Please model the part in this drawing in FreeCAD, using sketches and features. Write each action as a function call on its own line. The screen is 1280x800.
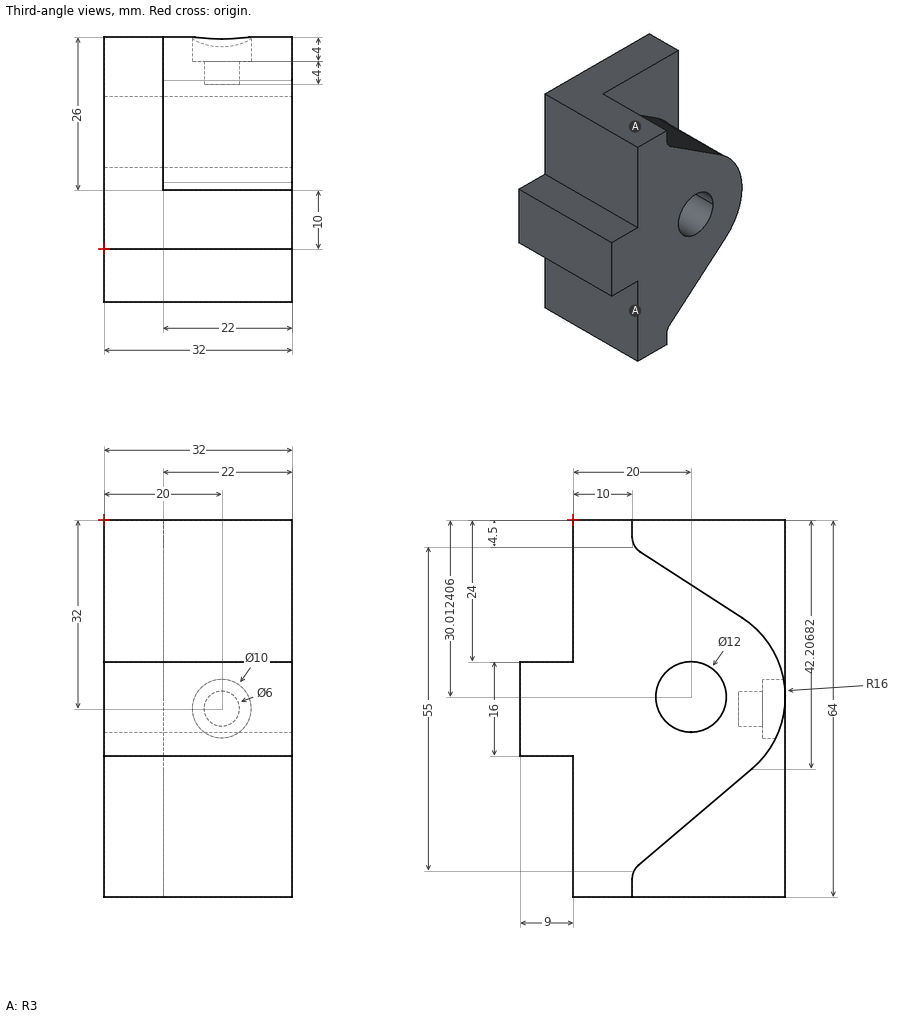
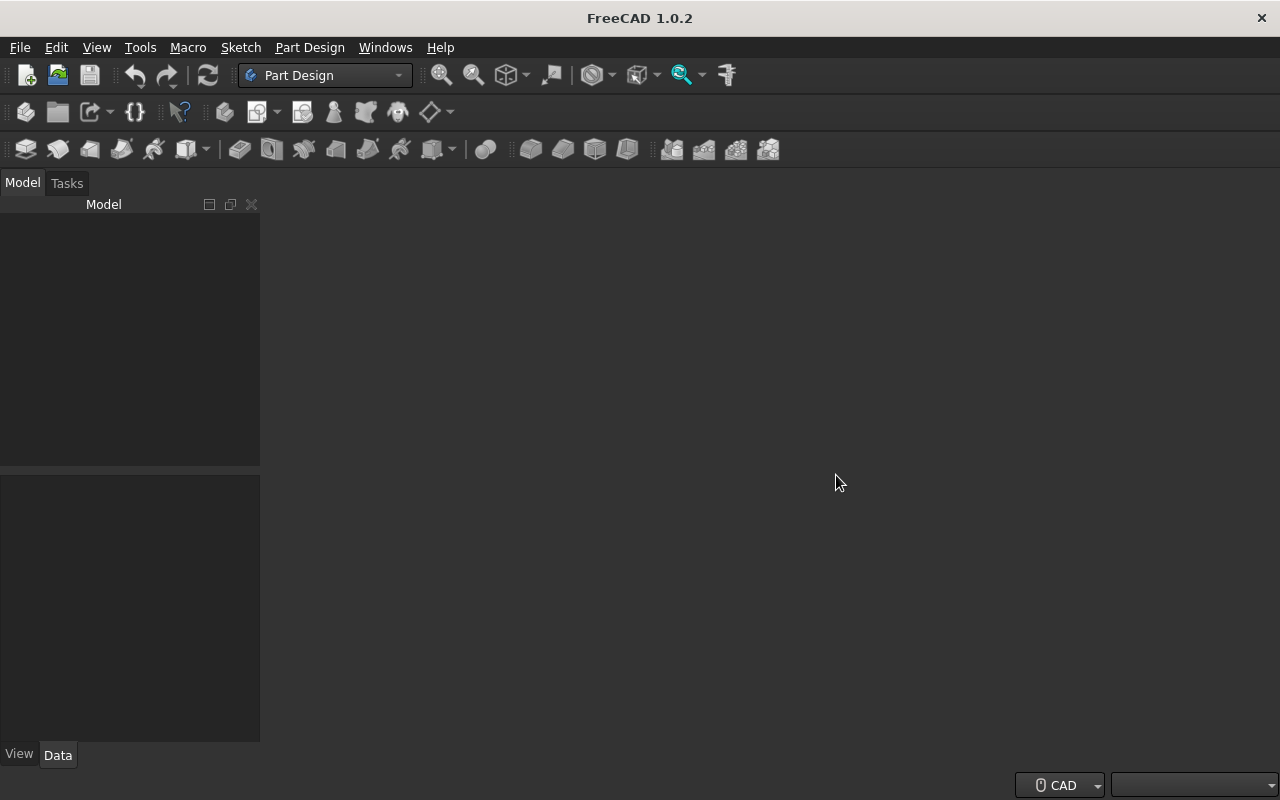
key(ctrl+n)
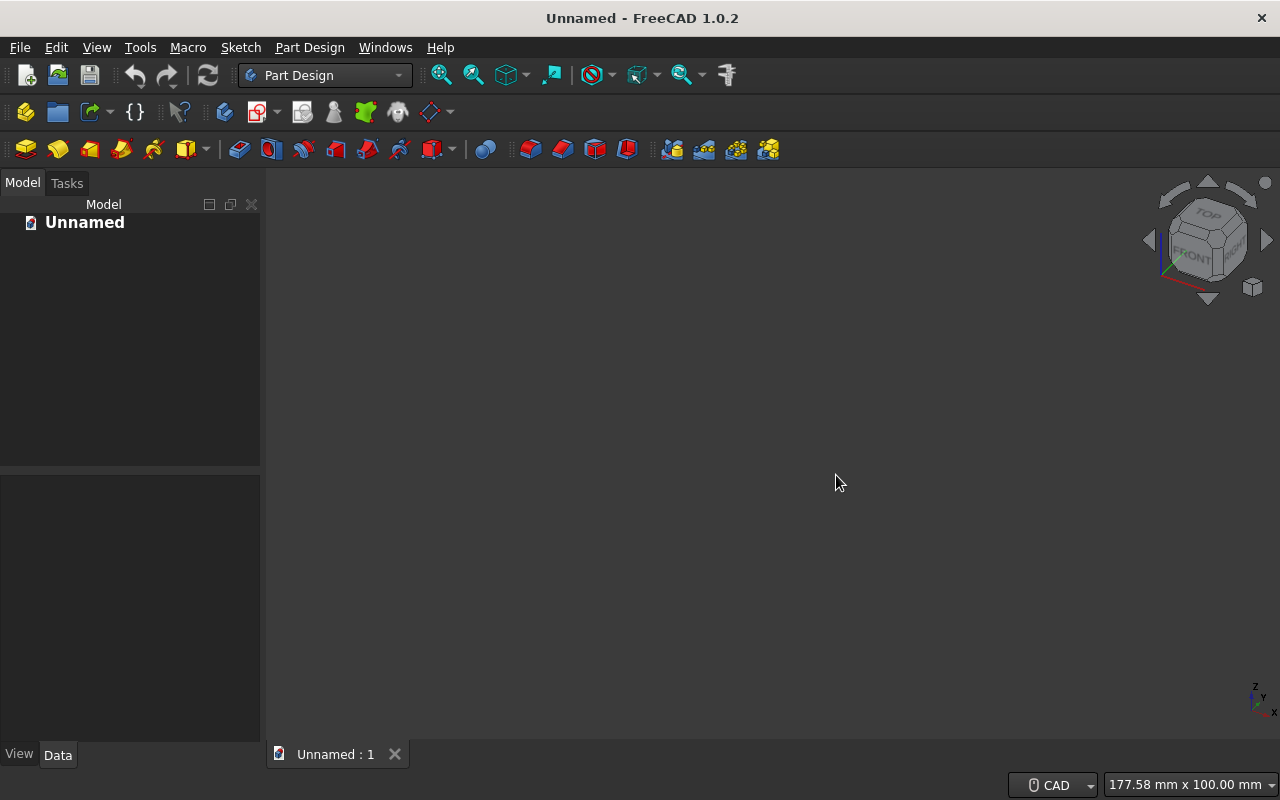
click(258, 112)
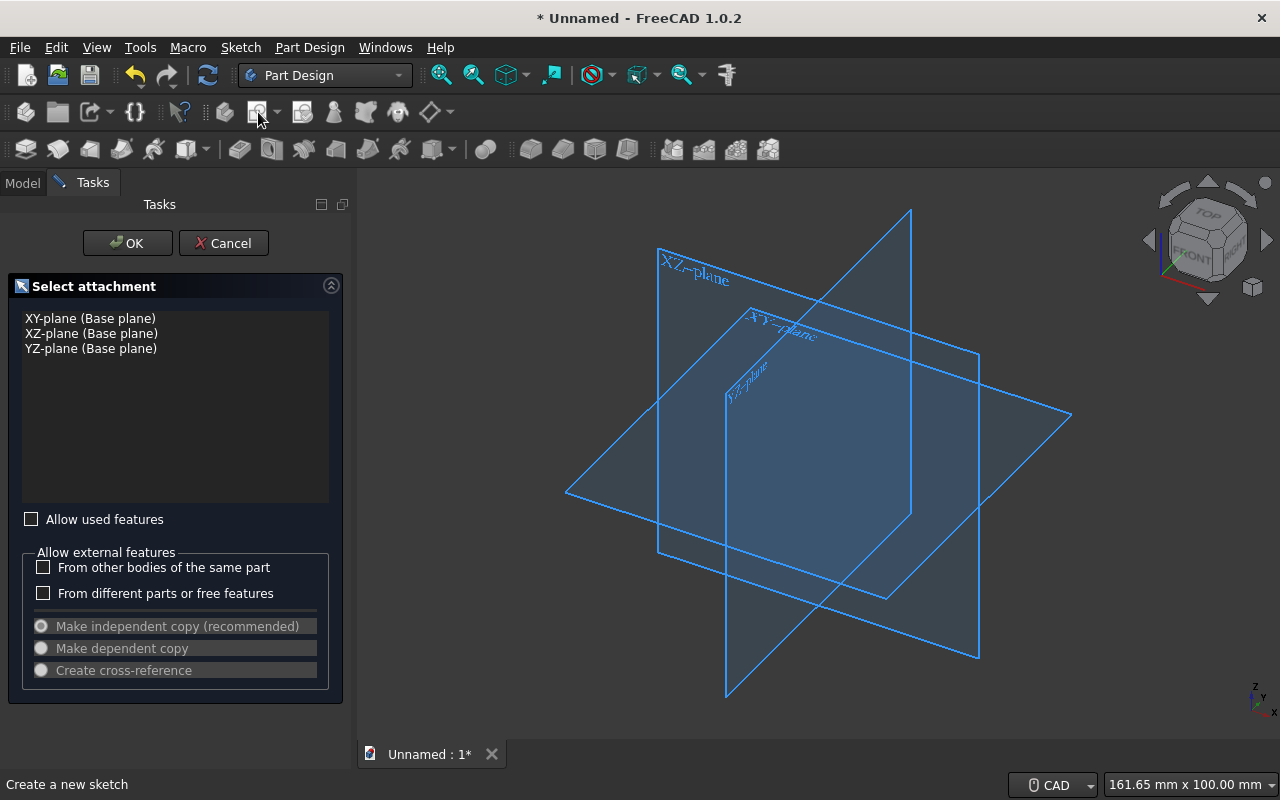
click(82, 318)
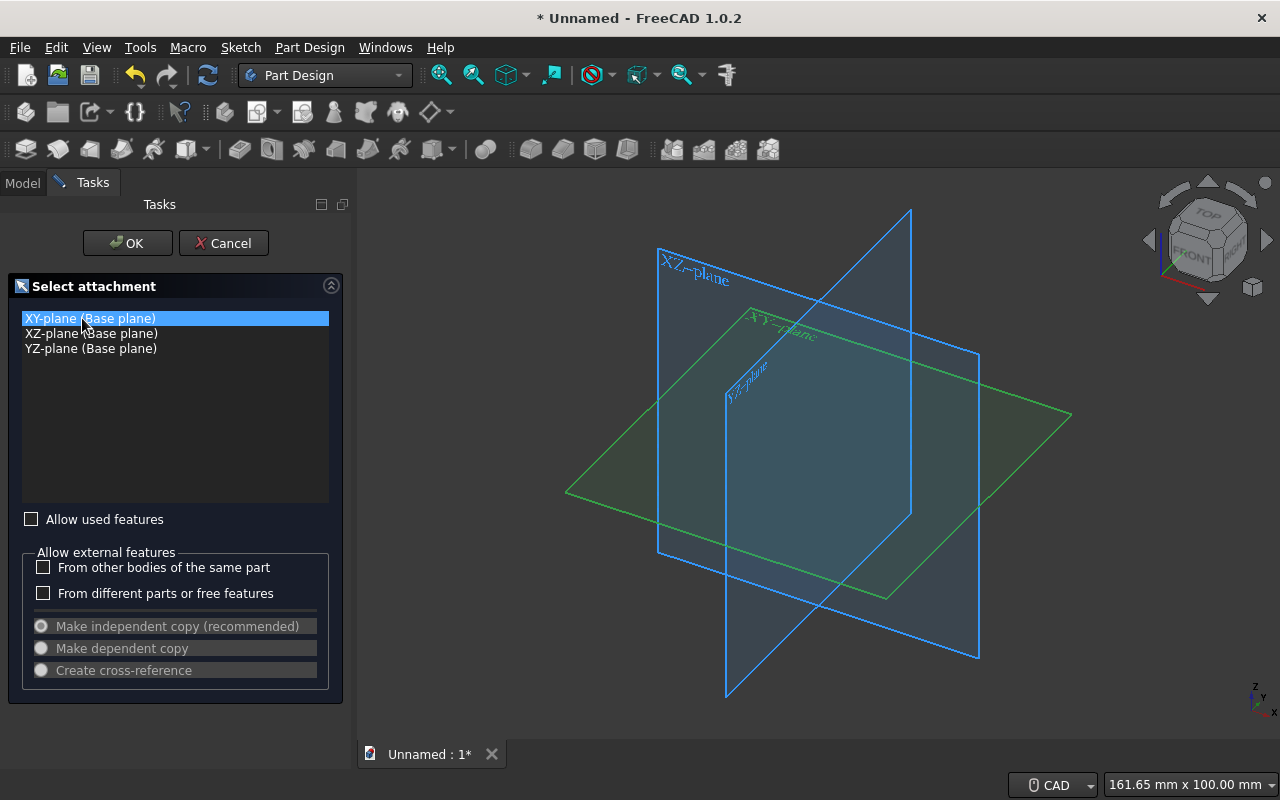
click(128, 243)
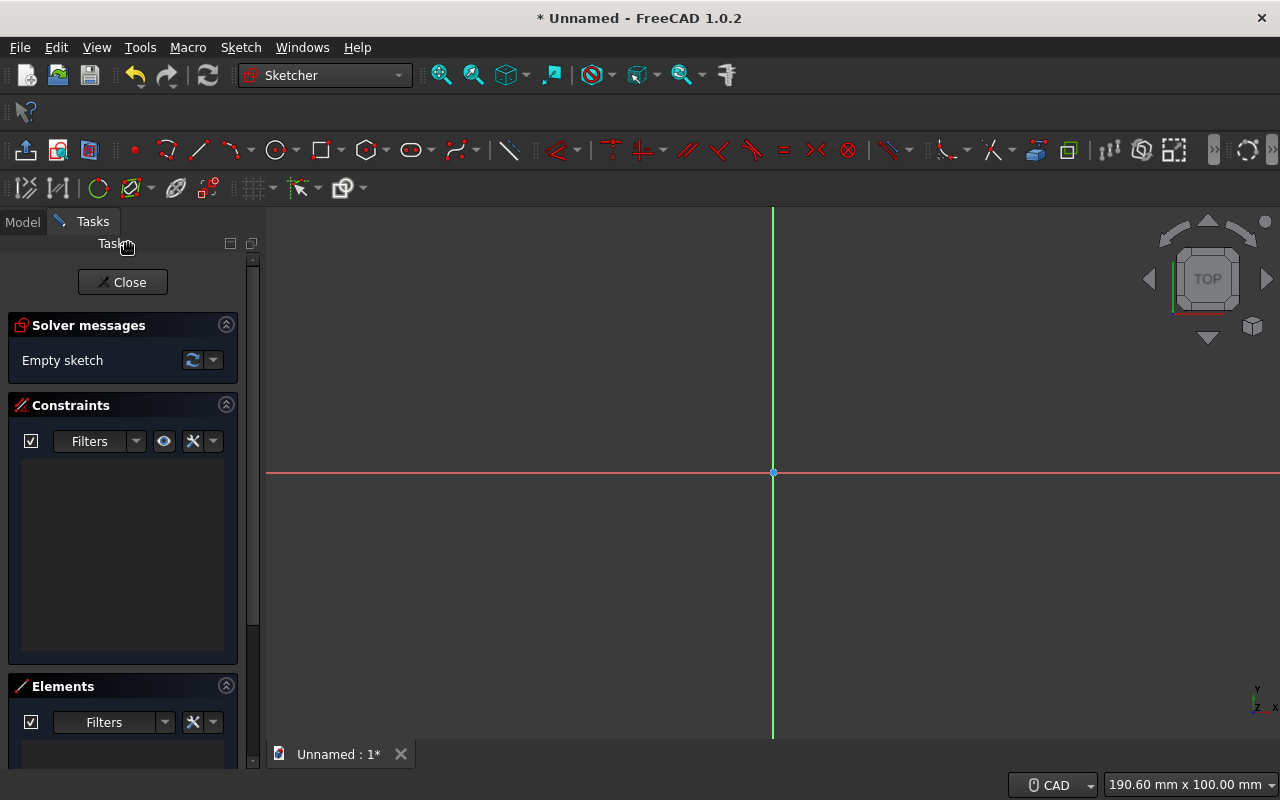
scroll(1045, 261, up, 3)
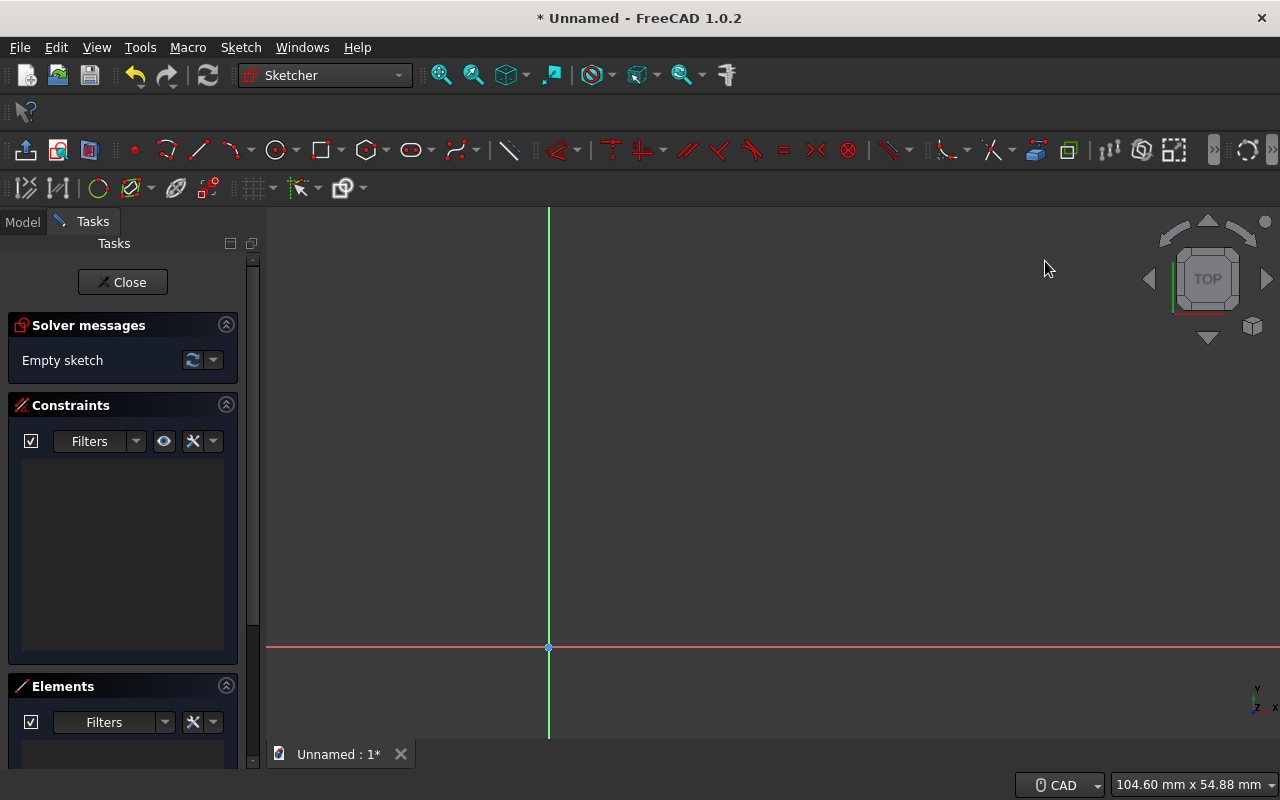
key(g)
key(m)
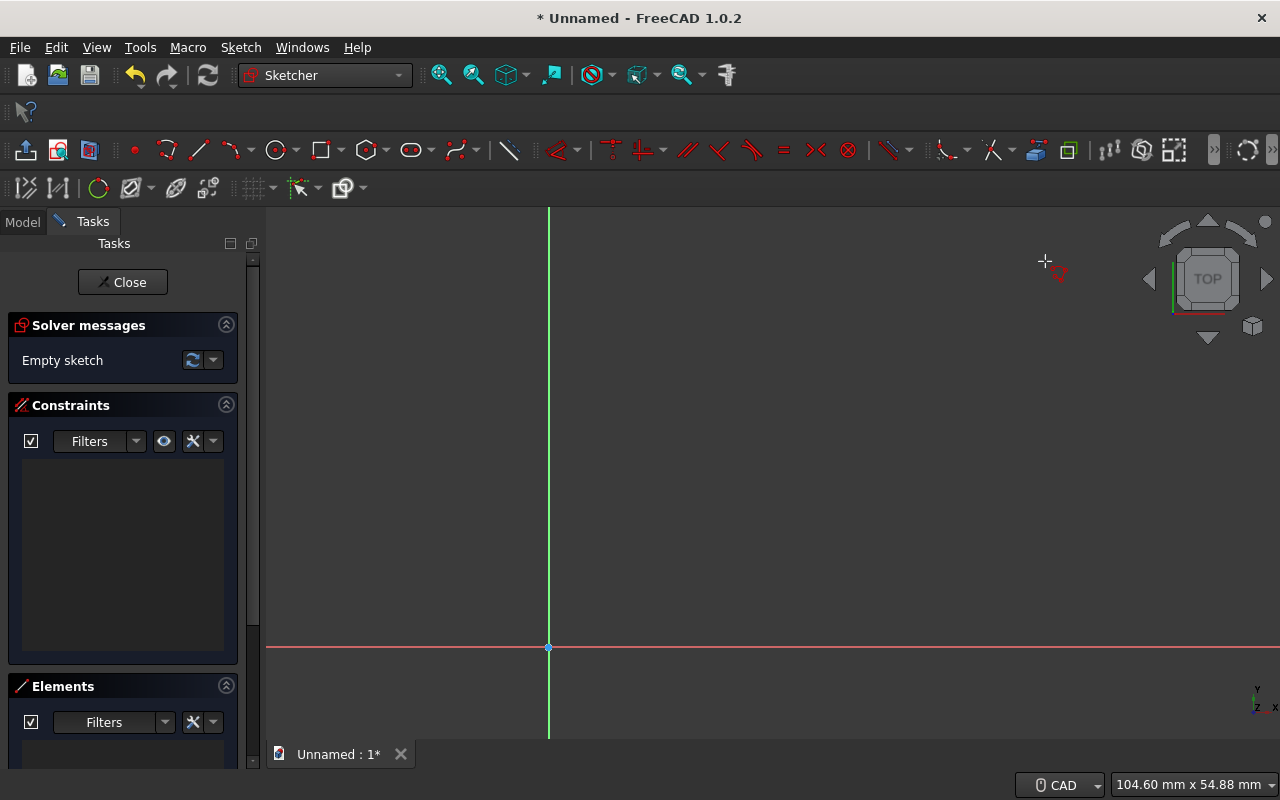
click(549, 647)
click(859, 638)
click(859, 550)
click(646, 550)
click(646, 298)
click(558, 298)
click(549, 647)
key(Escape)
key(Escape)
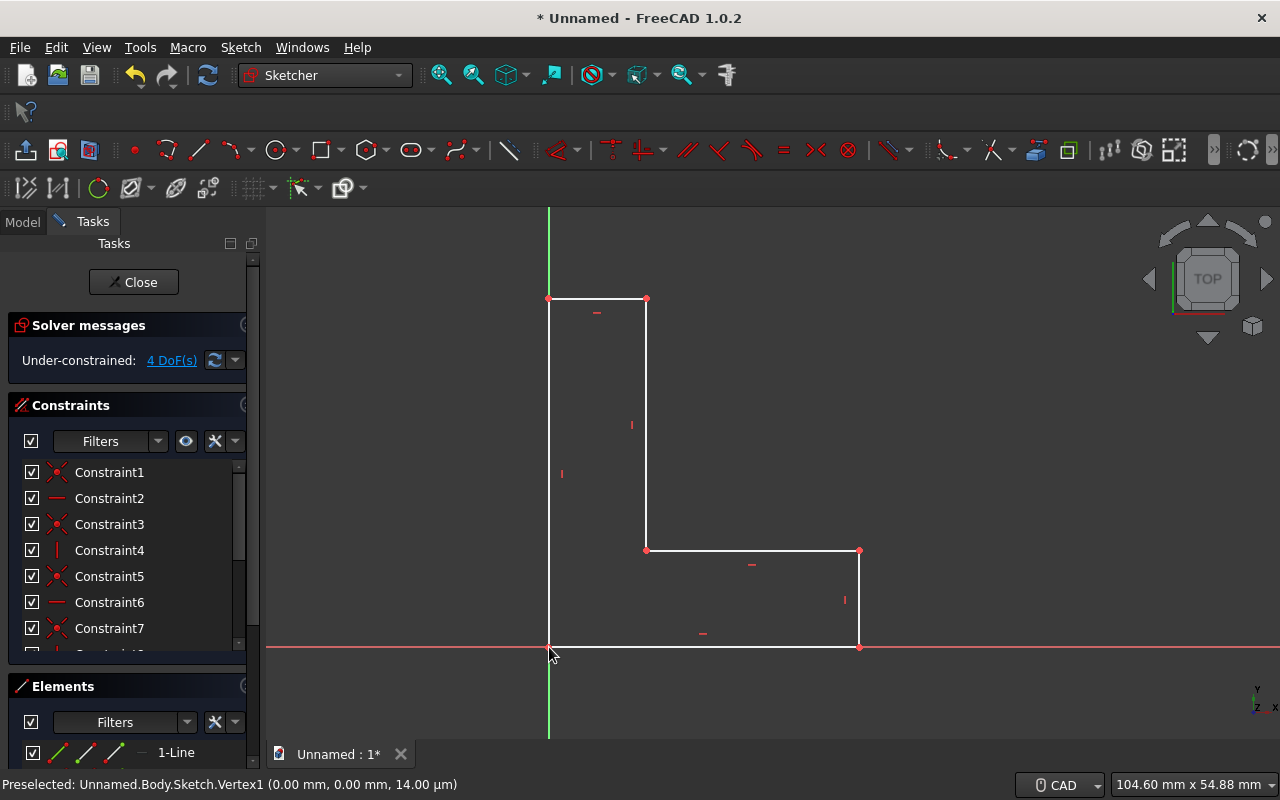
click(556, 150)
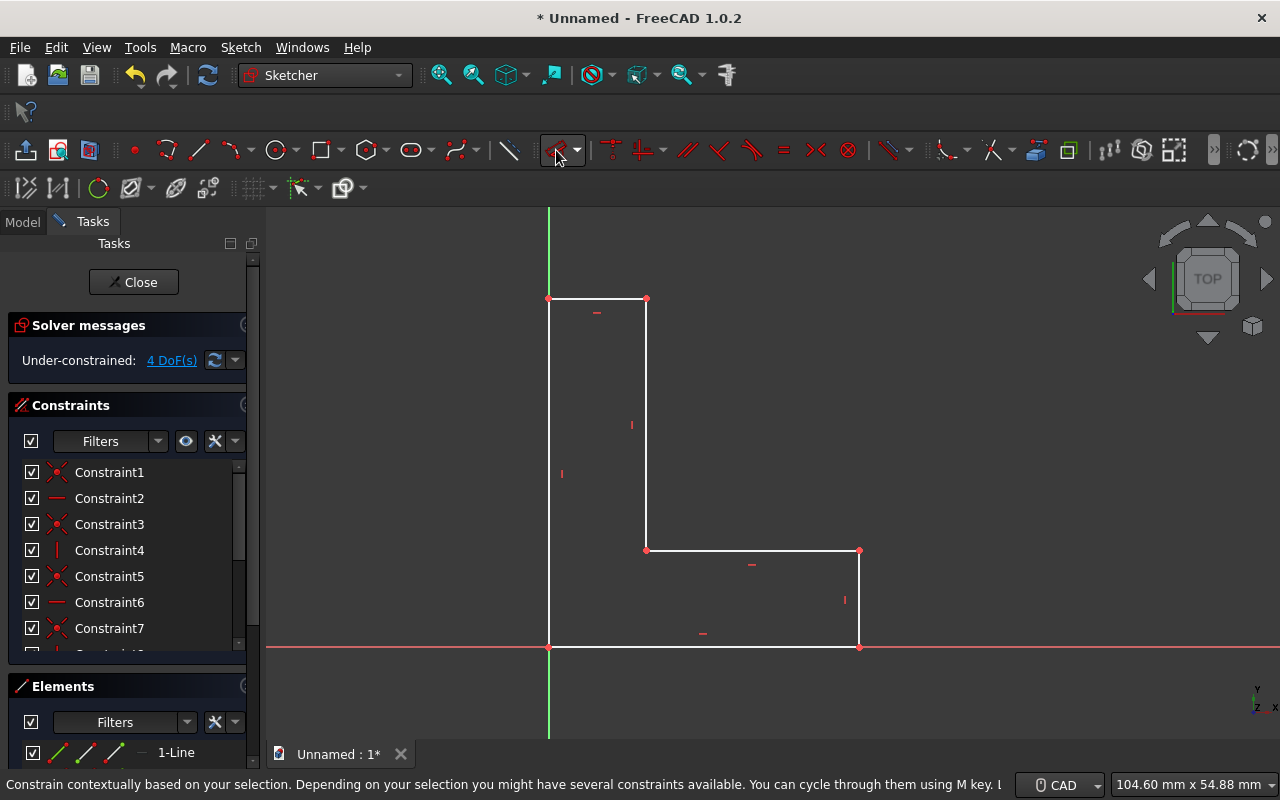
click(642, 647)
click(704, 681)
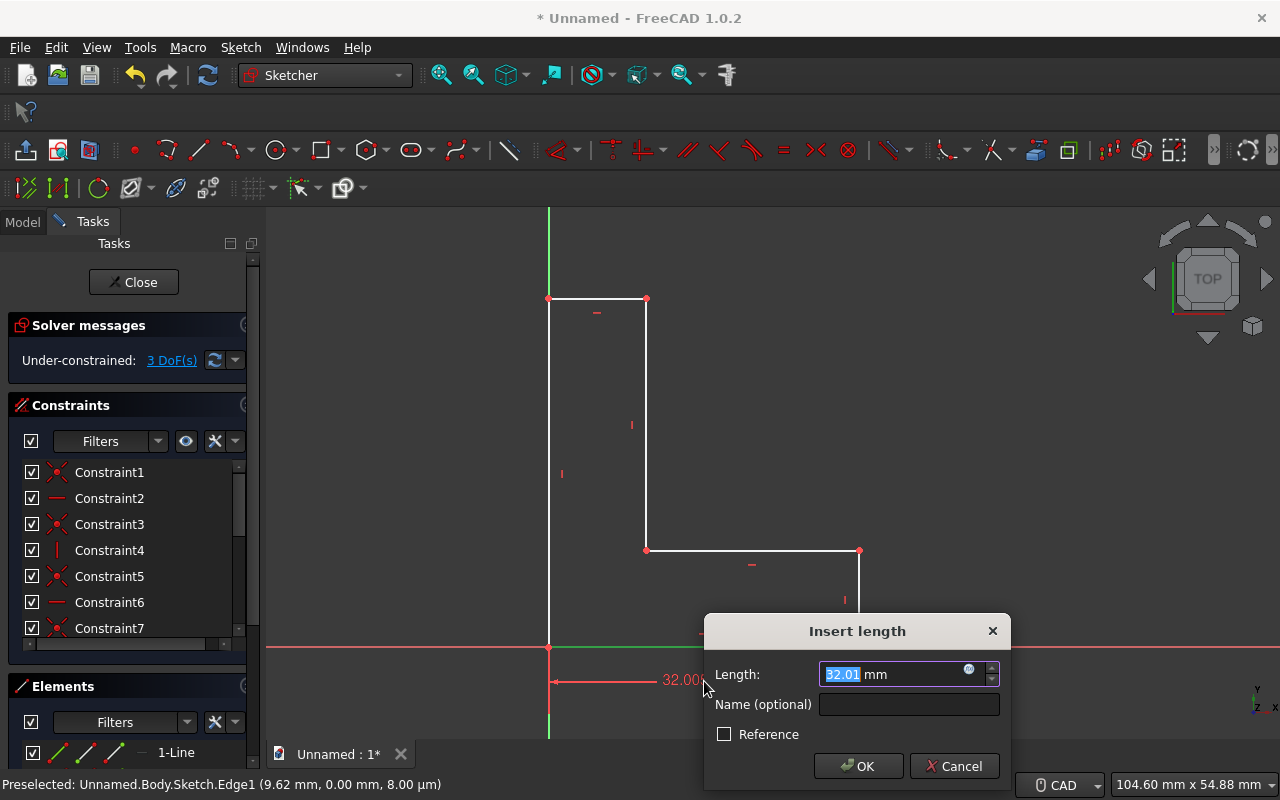
text(32)
key(Return)